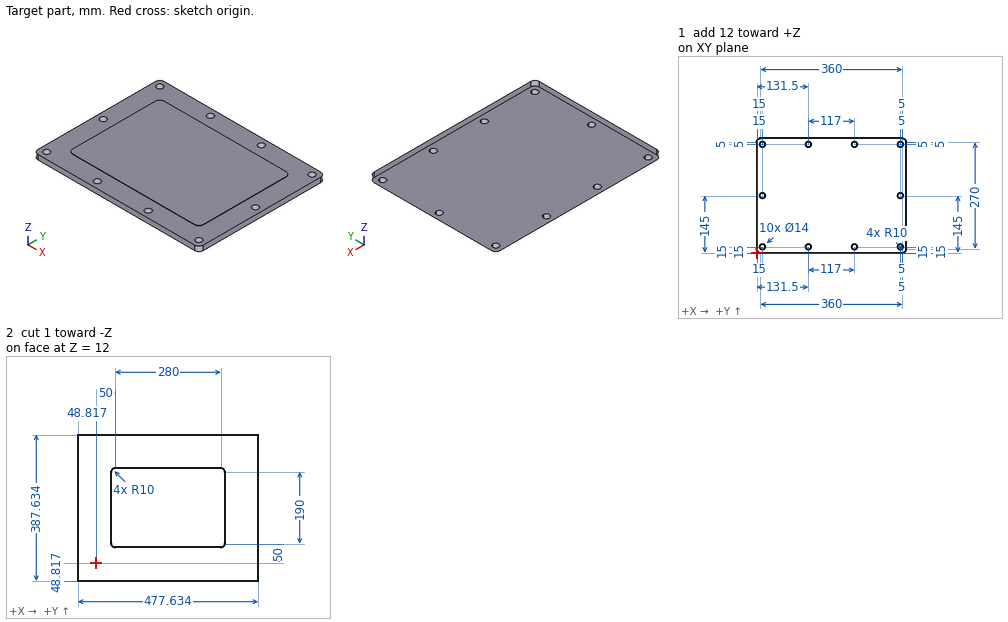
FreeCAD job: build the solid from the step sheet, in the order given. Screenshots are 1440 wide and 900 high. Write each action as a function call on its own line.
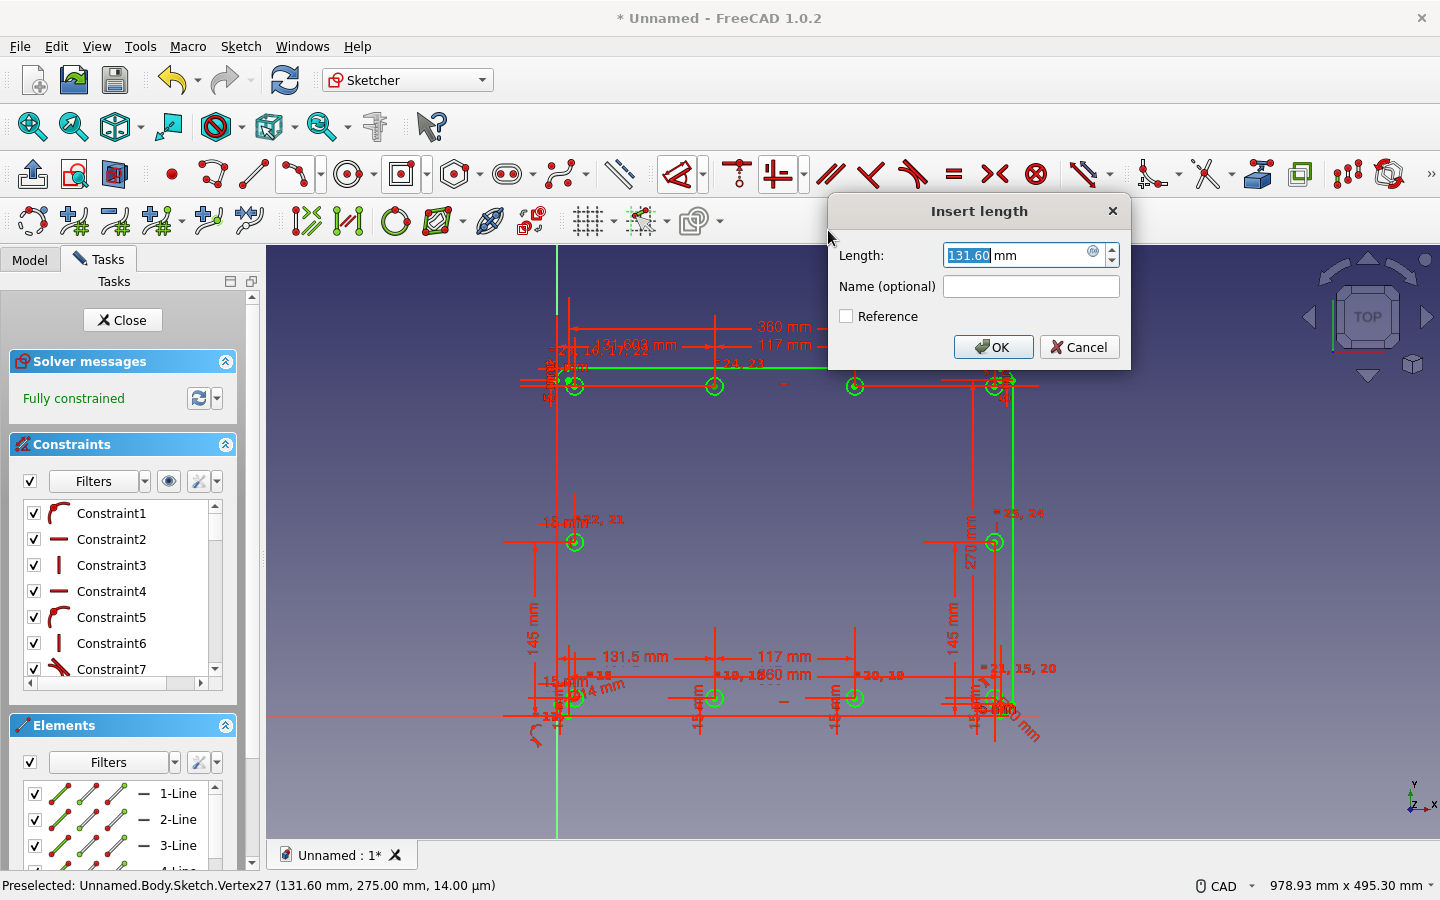
text(131.5)
key(Return)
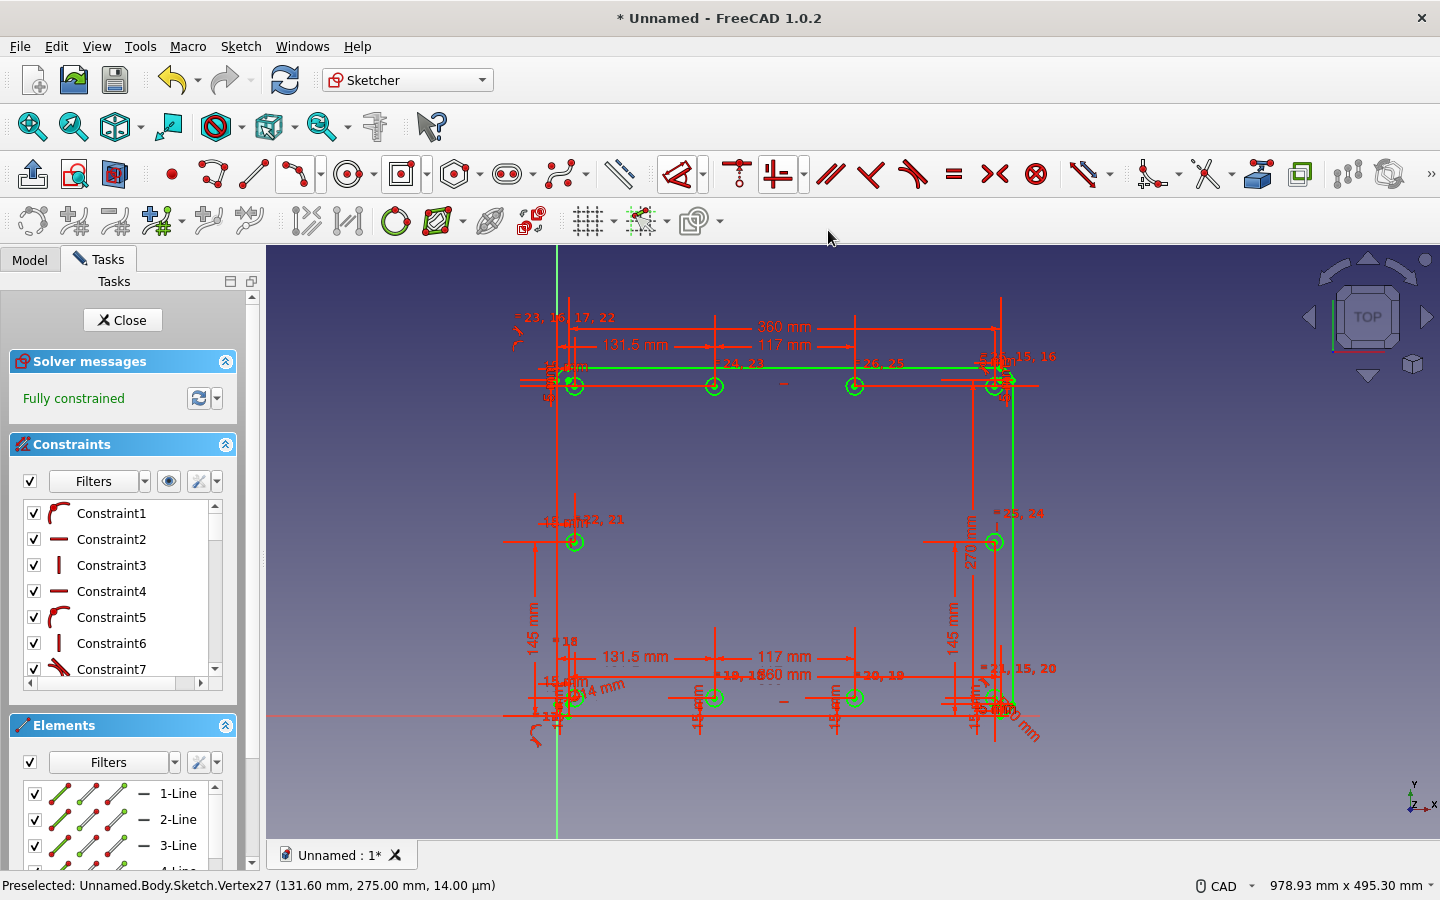
click(123, 320)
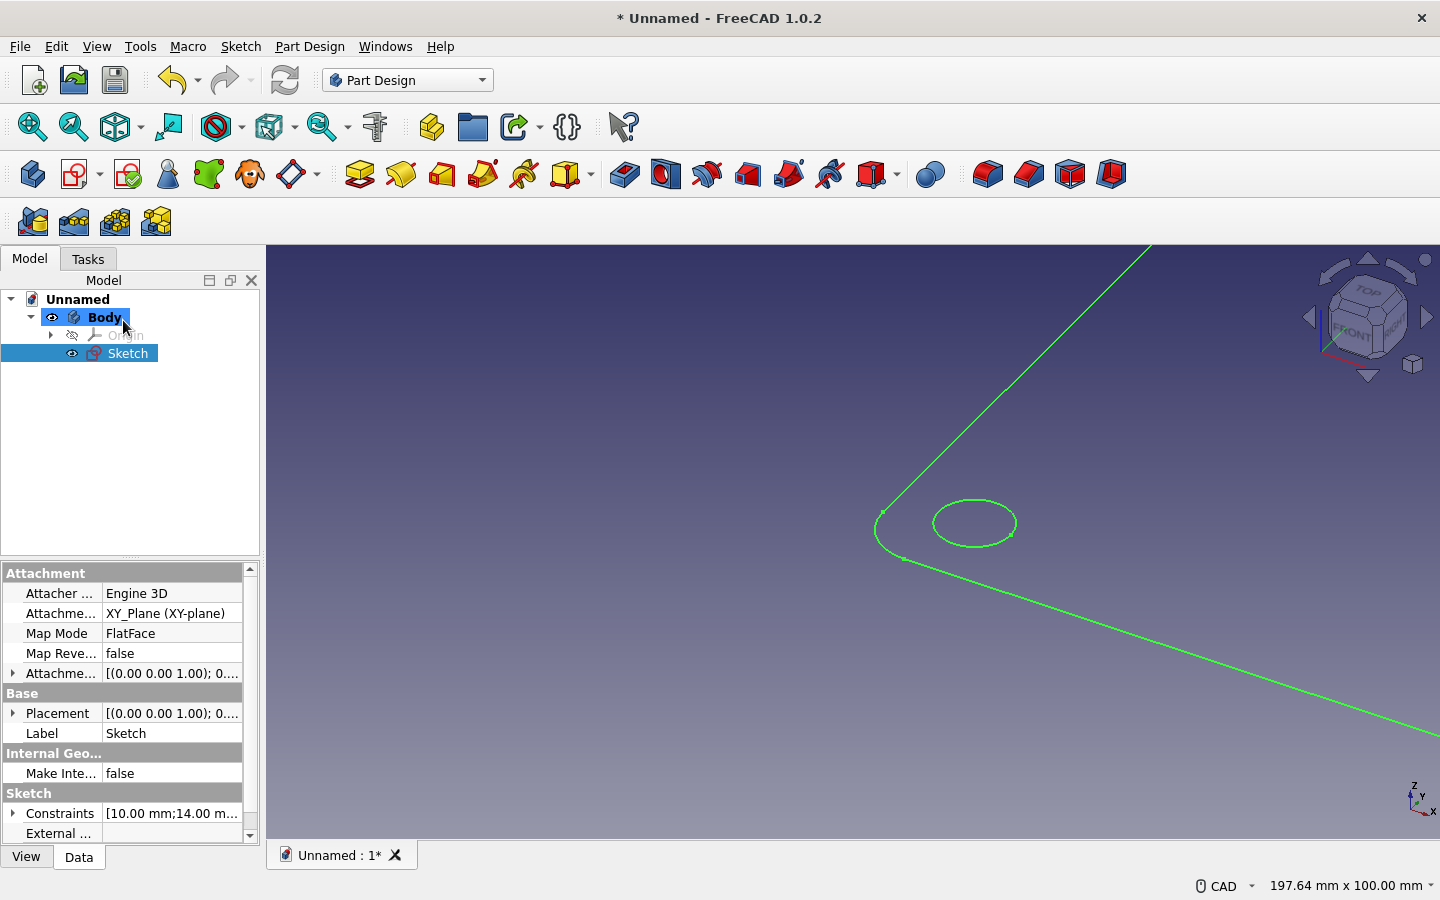
click(360, 174)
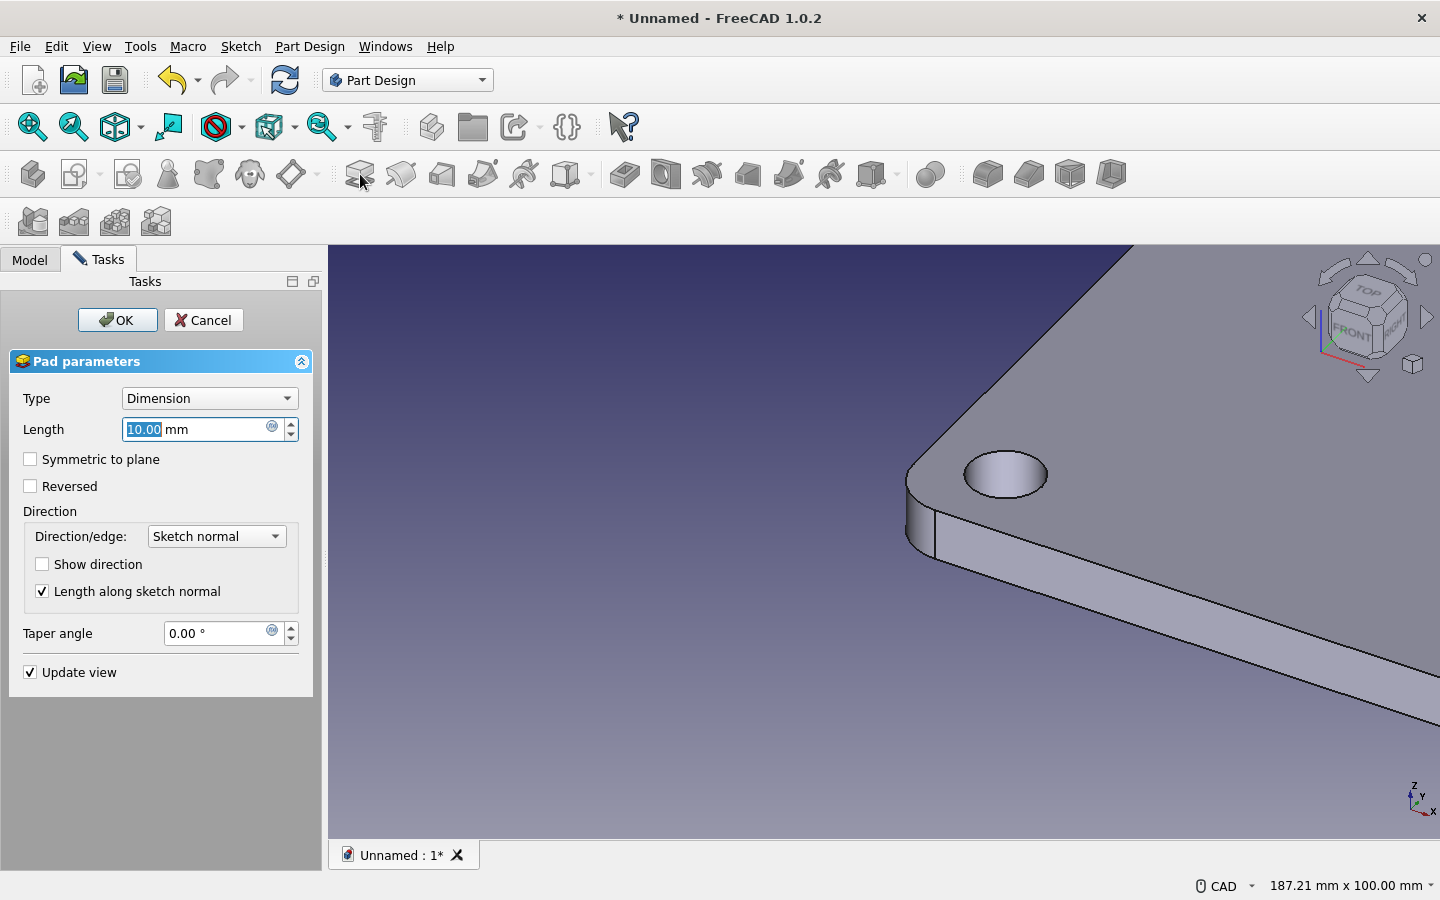
text(12)
key(Tab)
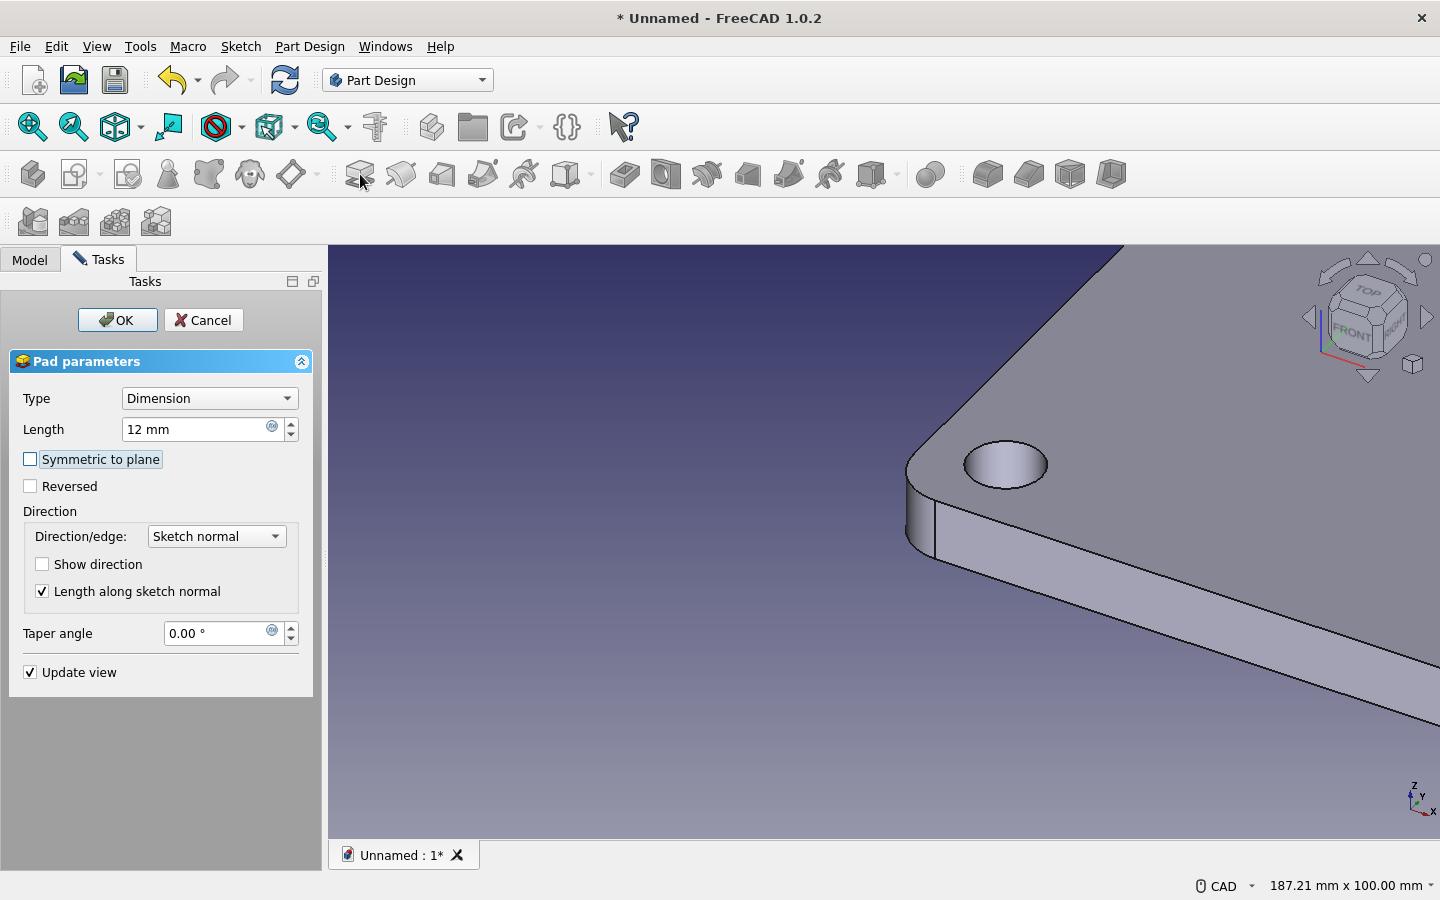
click(118, 320)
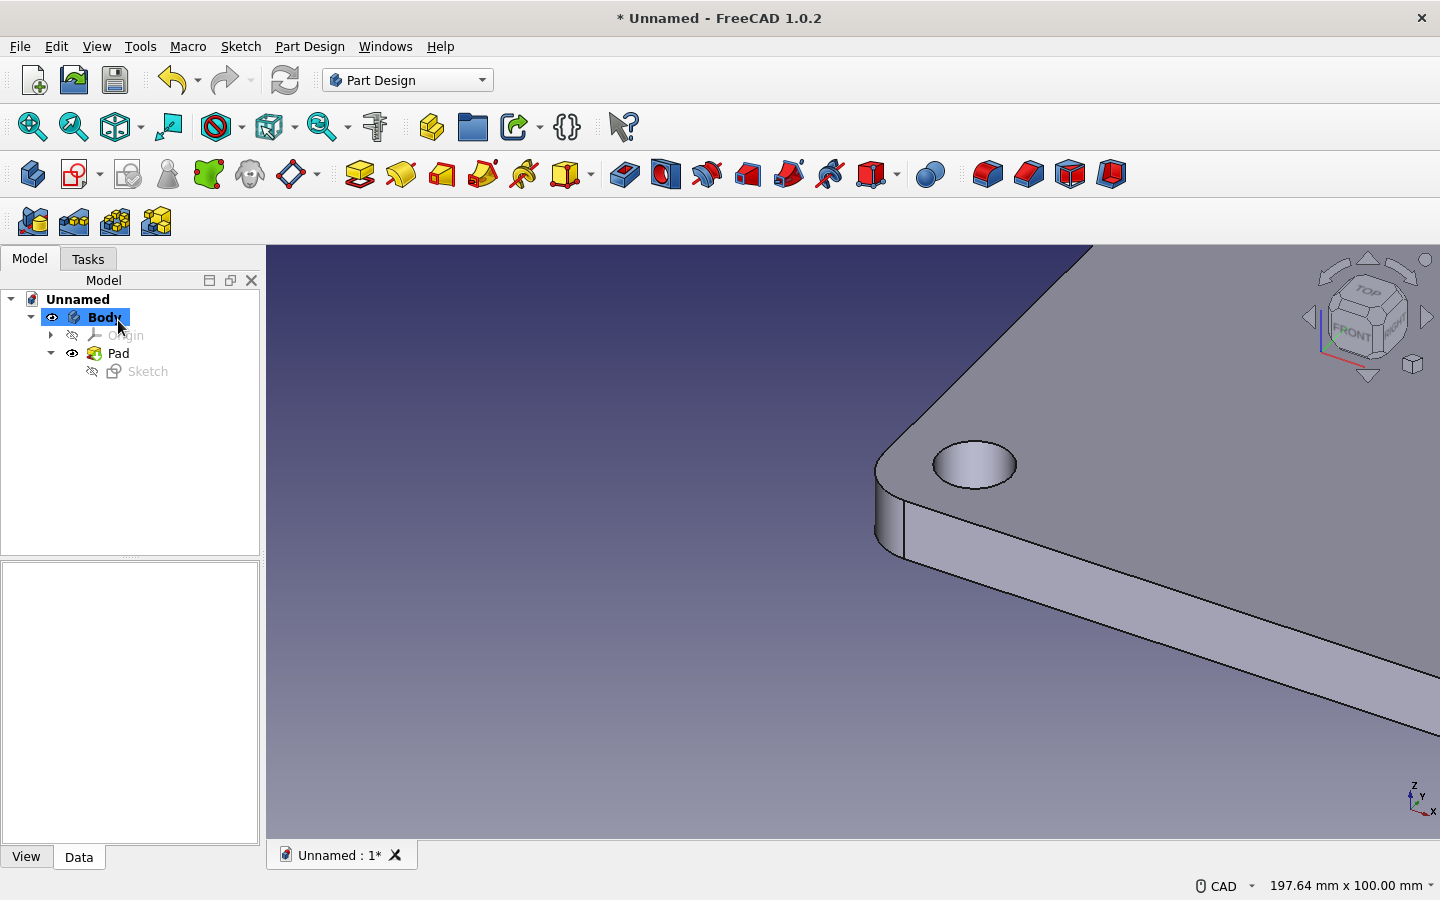
click(33, 128)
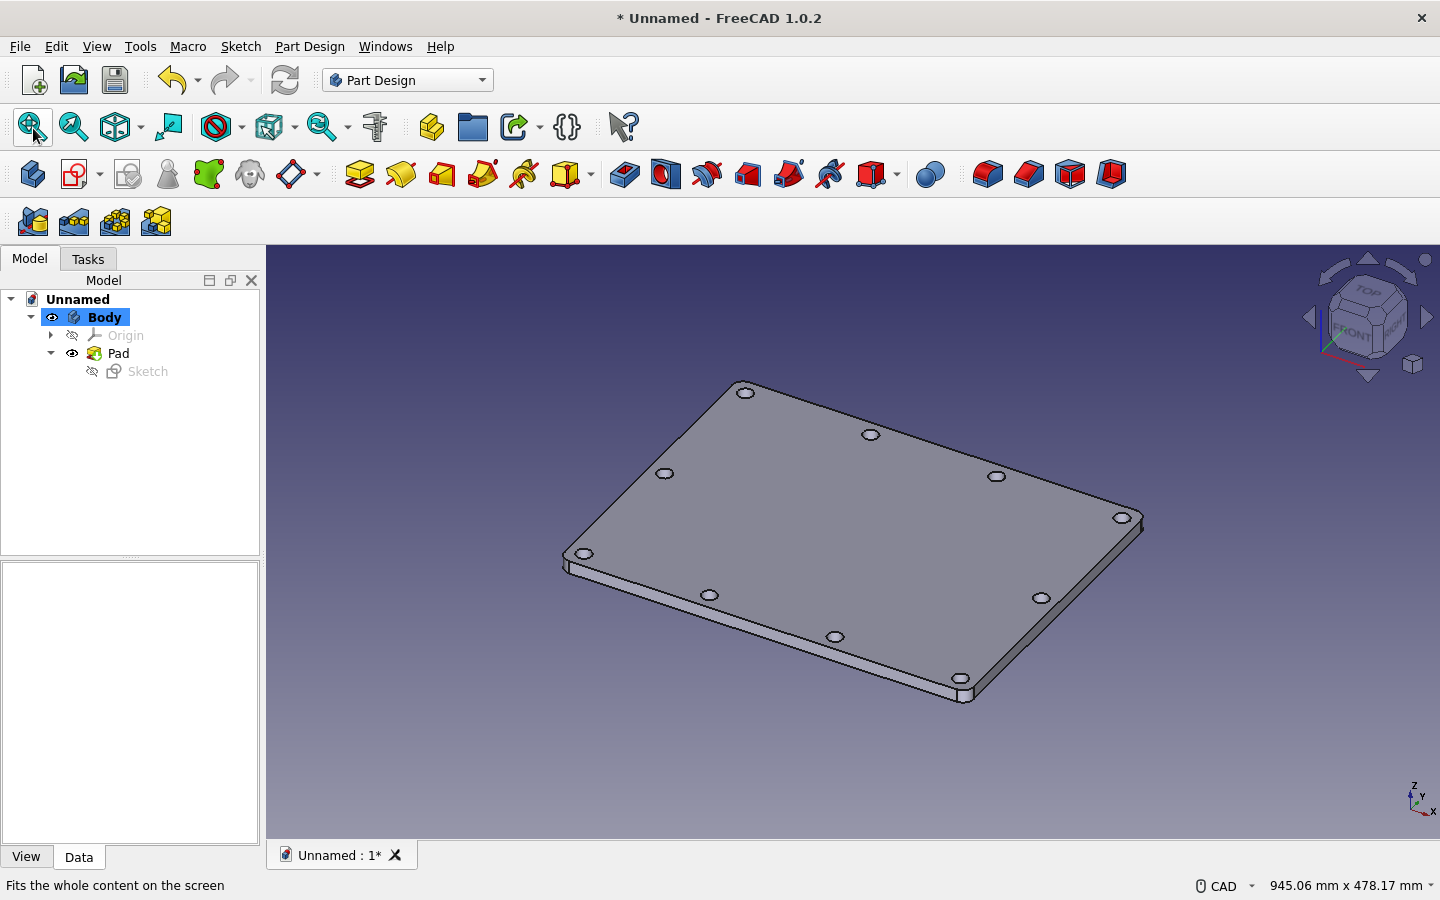
click(853, 535)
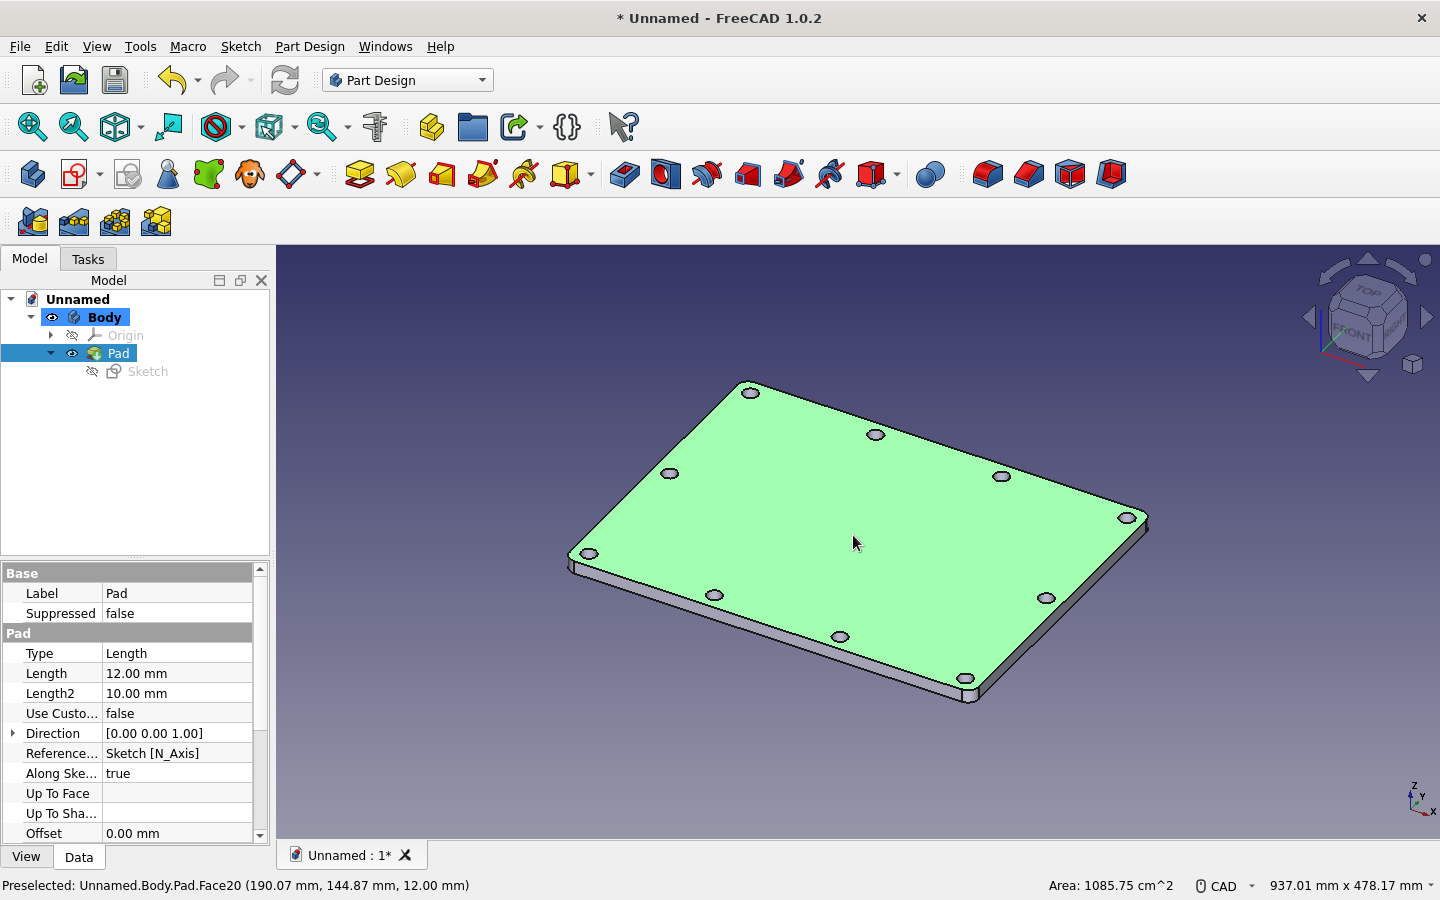
click(74, 174)